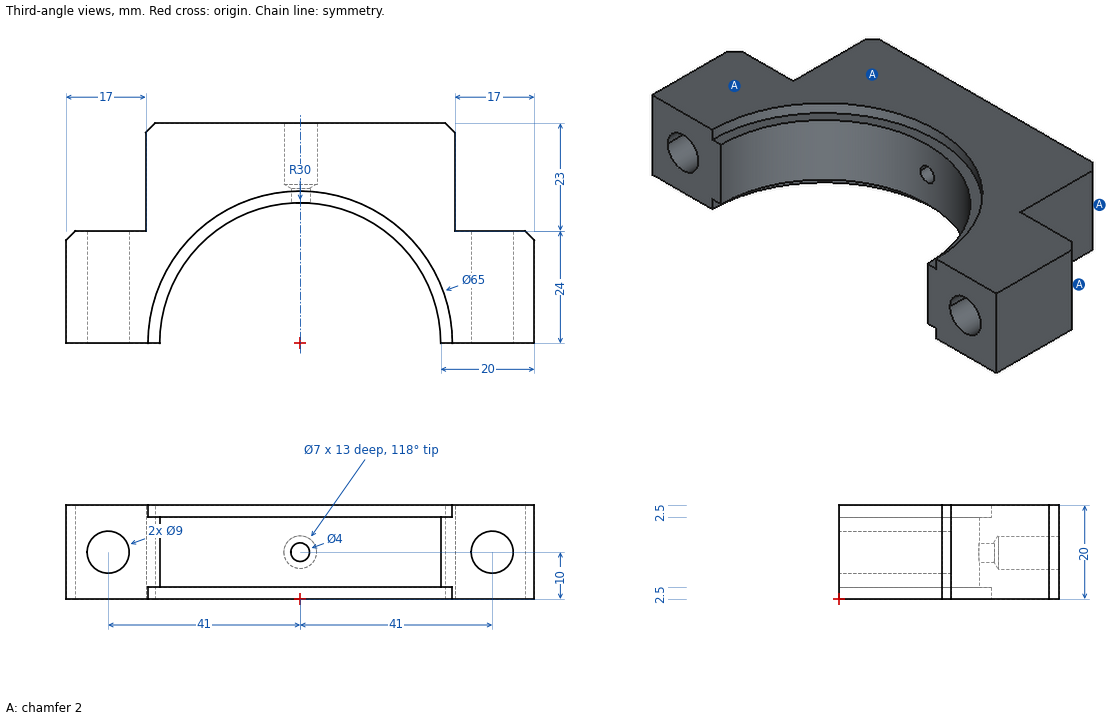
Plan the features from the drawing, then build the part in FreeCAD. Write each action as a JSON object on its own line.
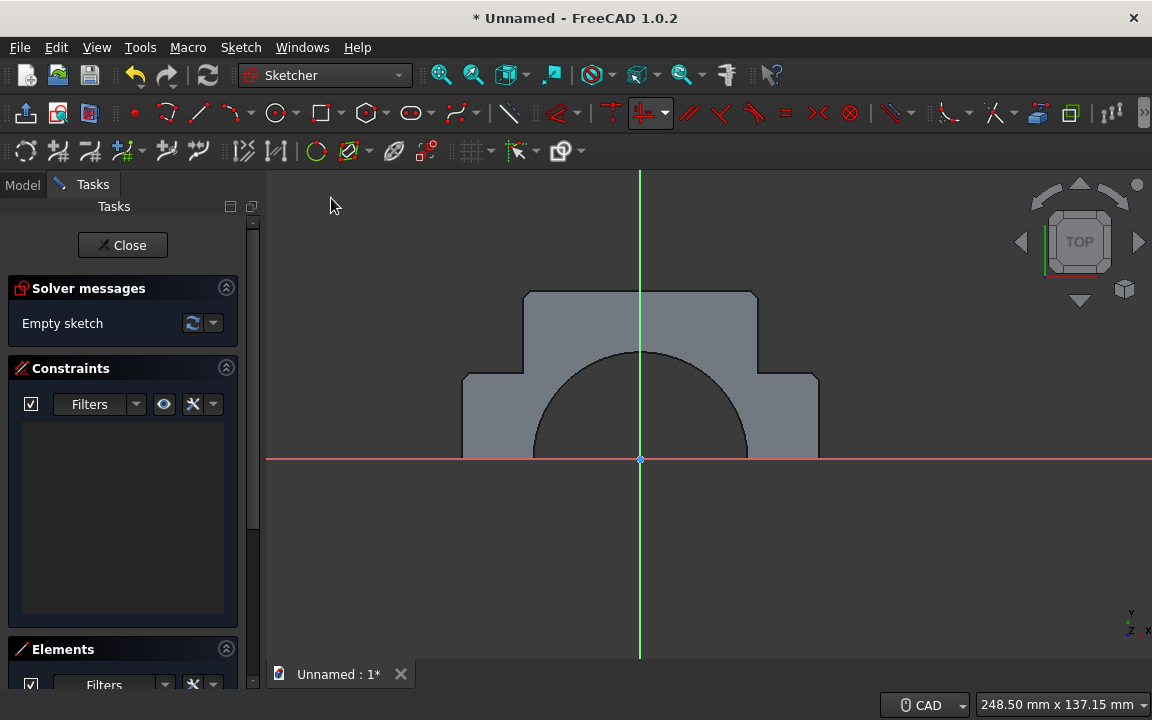
{"action": "left_click", "coordinate": [276, 114]}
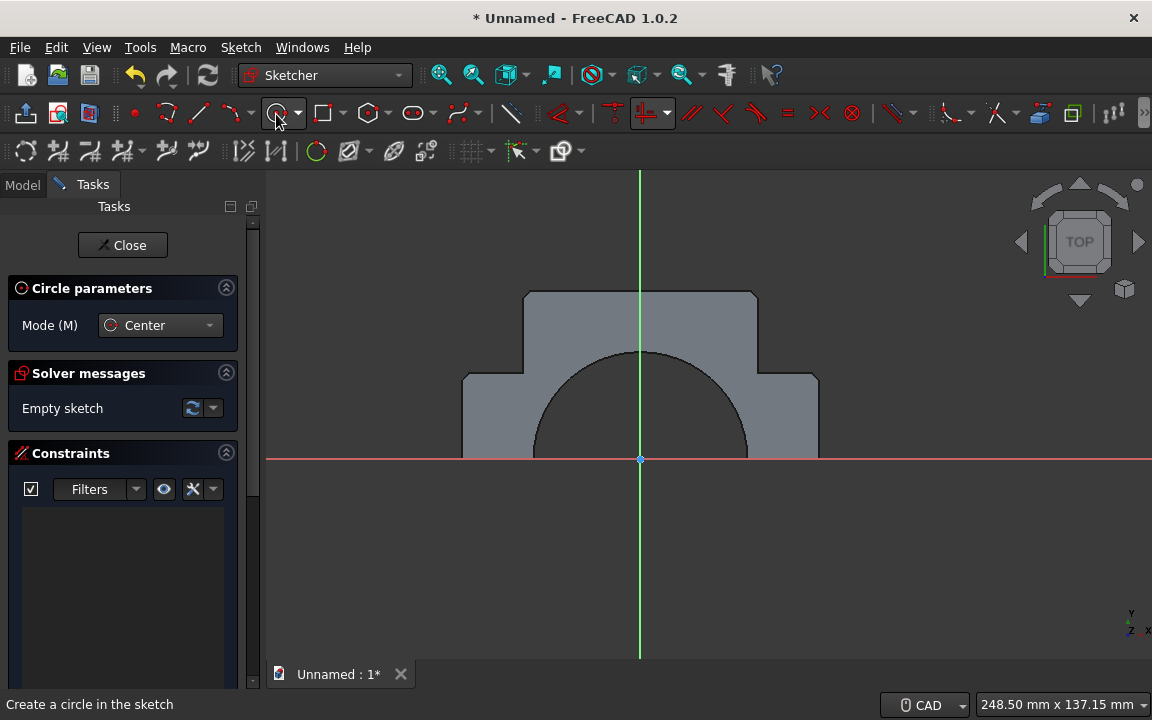
{"action": "left_click", "coordinate": [640, 459]}
{"action": "mouse_move", "coordinate": [722, 377]}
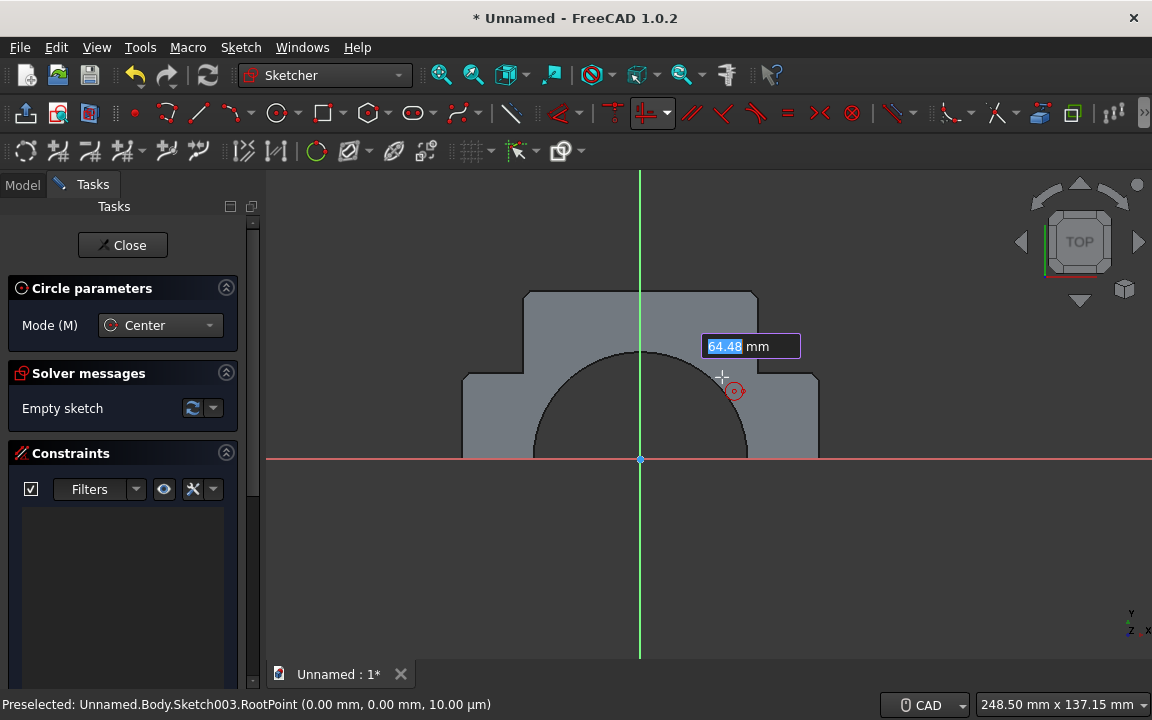
{"action": "type", "text": "65"}
{"action": "key", "text": "Return"}
{"action": "key", "text": "Escape"}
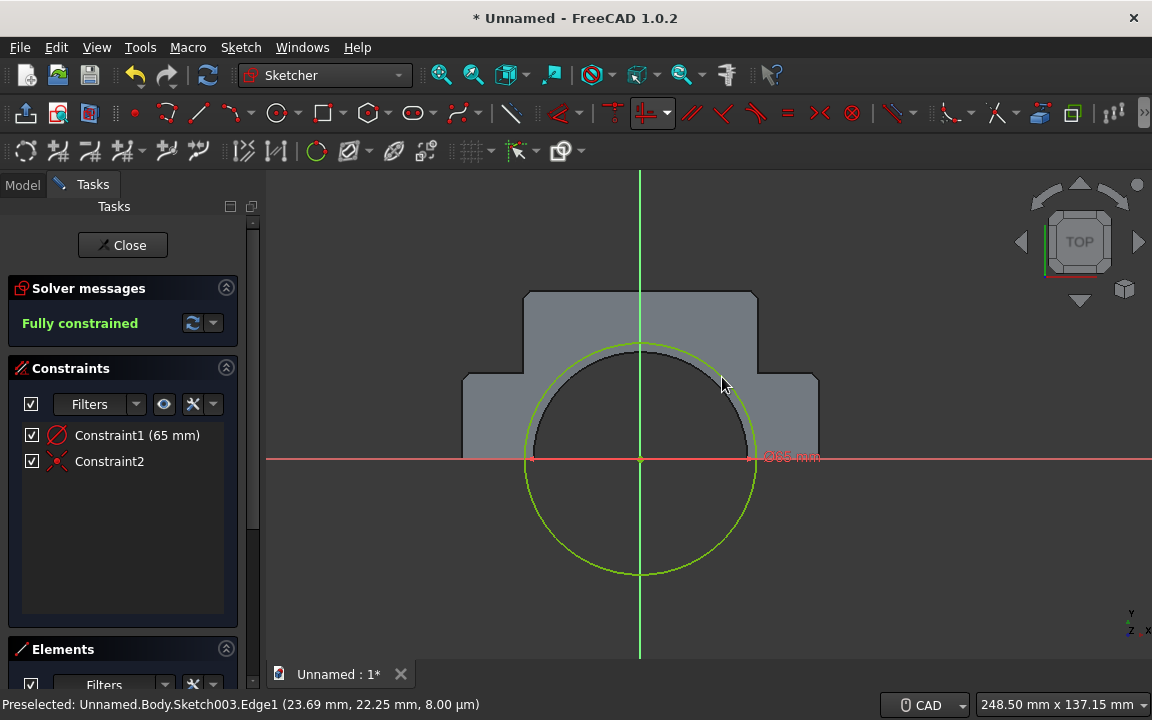
{"action": "left_click", "coordinate": [123, 245]}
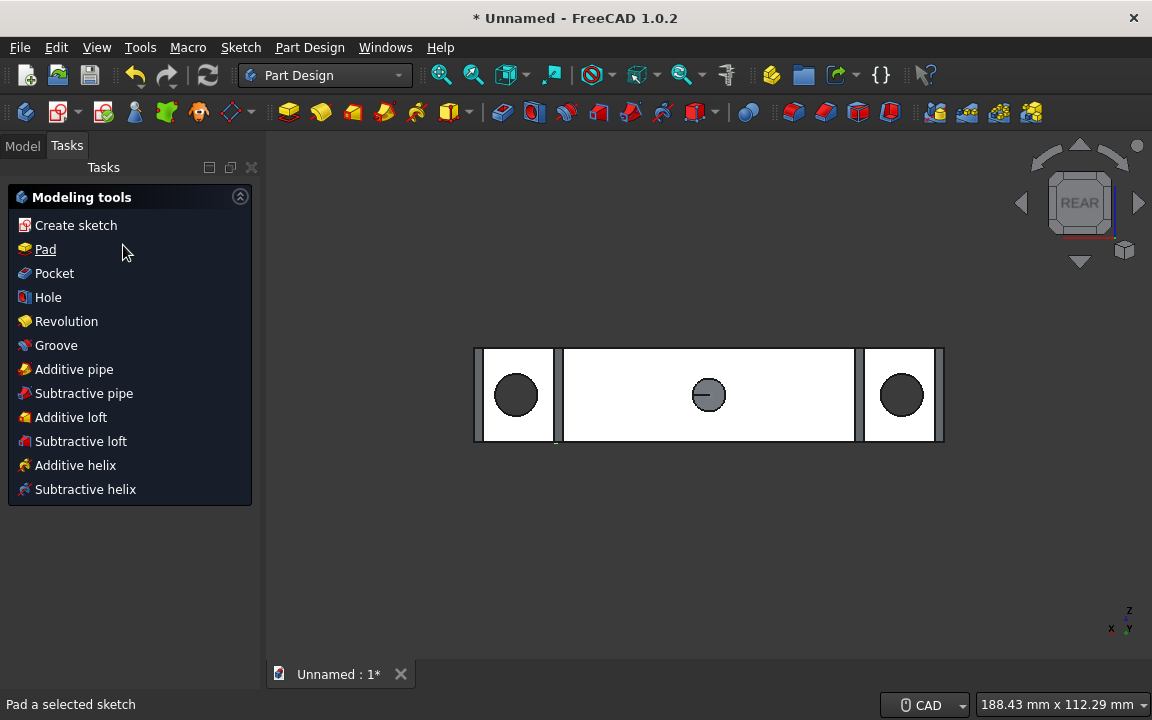
{"action": "left_click", "coordinate": [504, 112]}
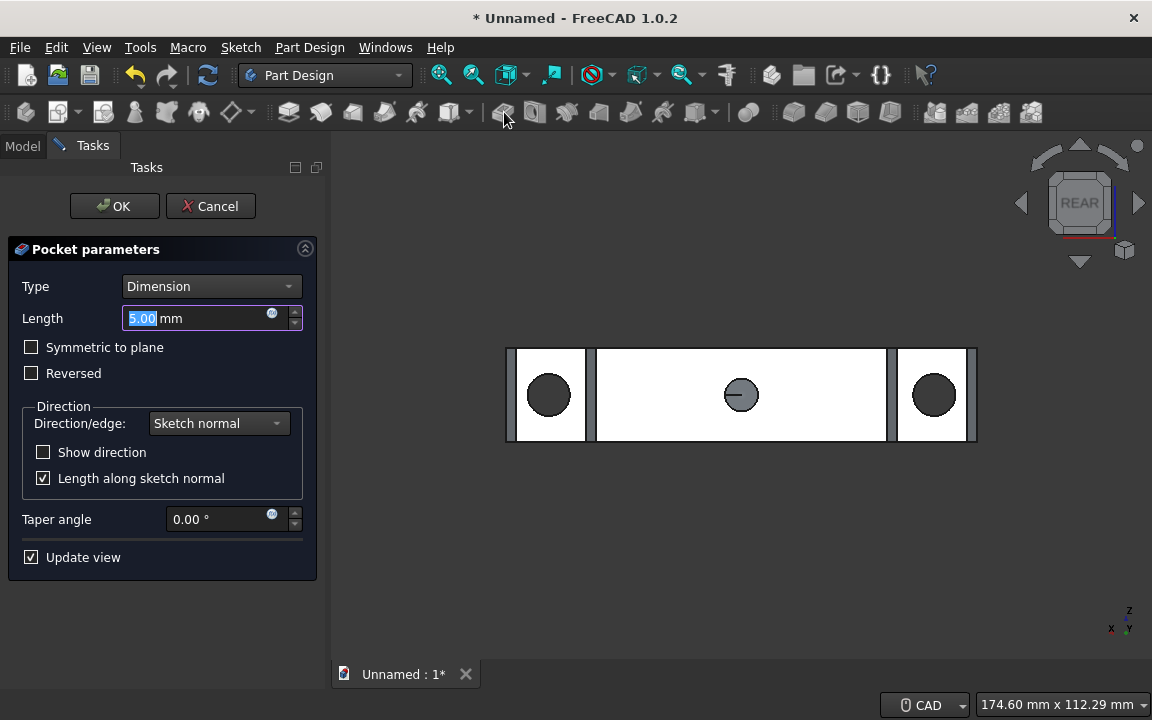
{"action": "type", "text": "2.5"}
{"action": "key", "text": "Tab"}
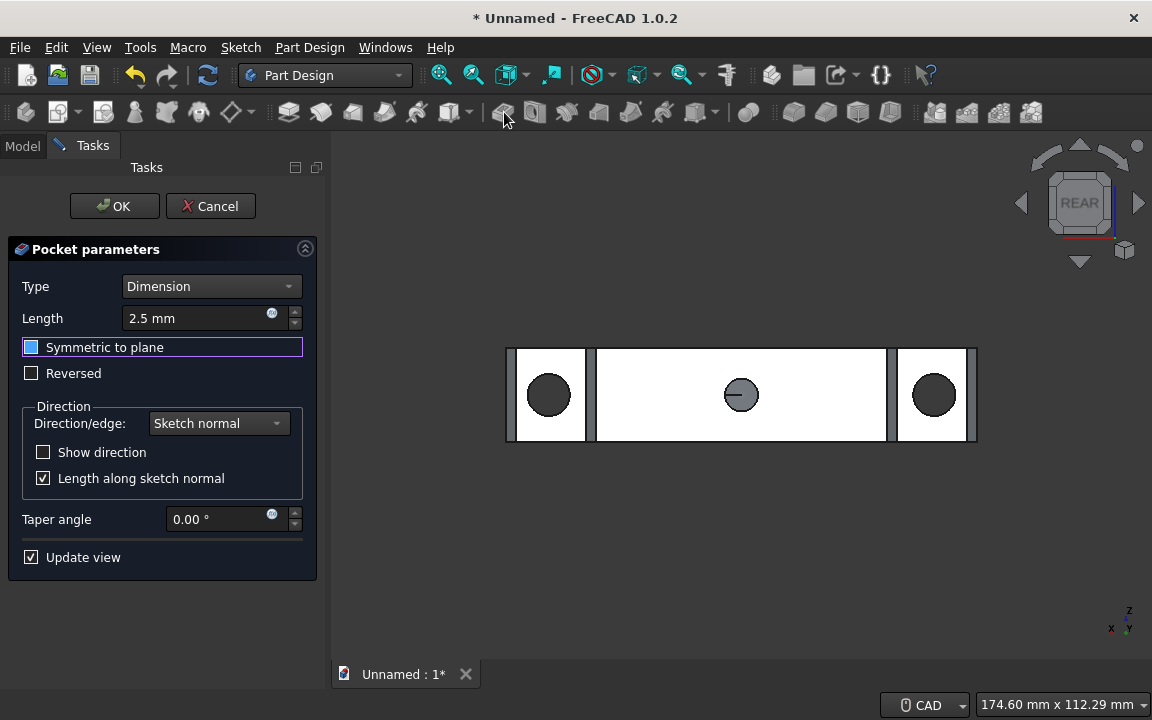
{"action": "left_click", "coordinate": [30, 373]}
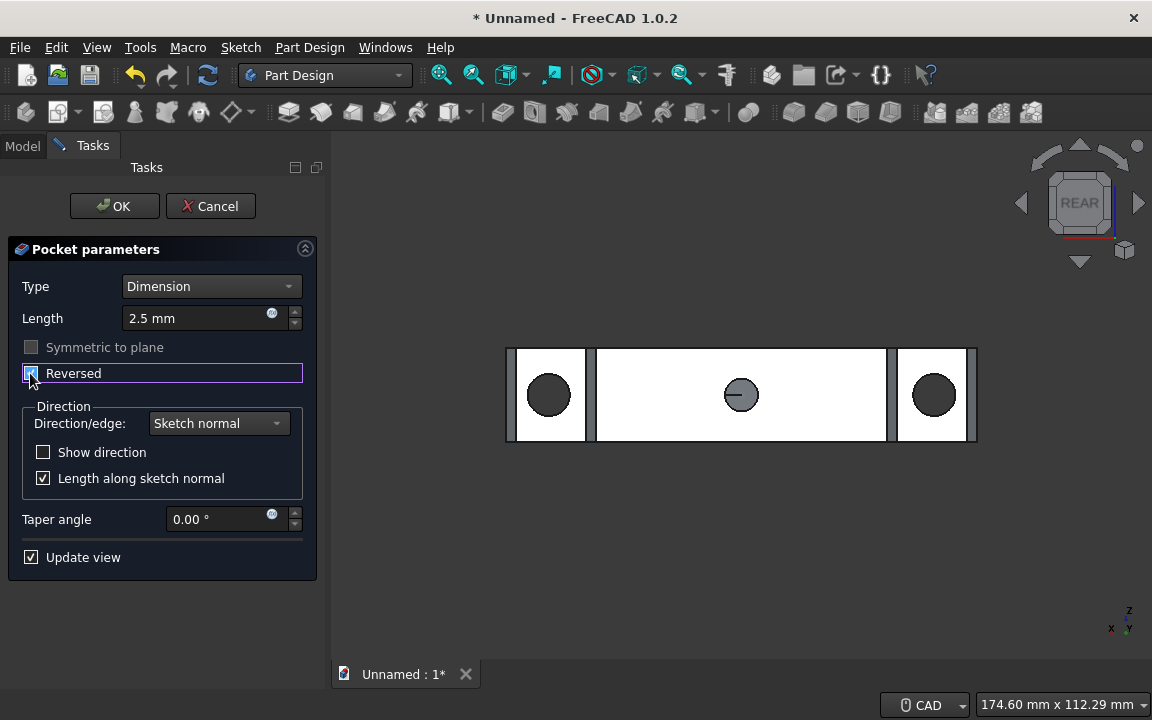
{"action": "left_click", "coordinate": [115, 206]}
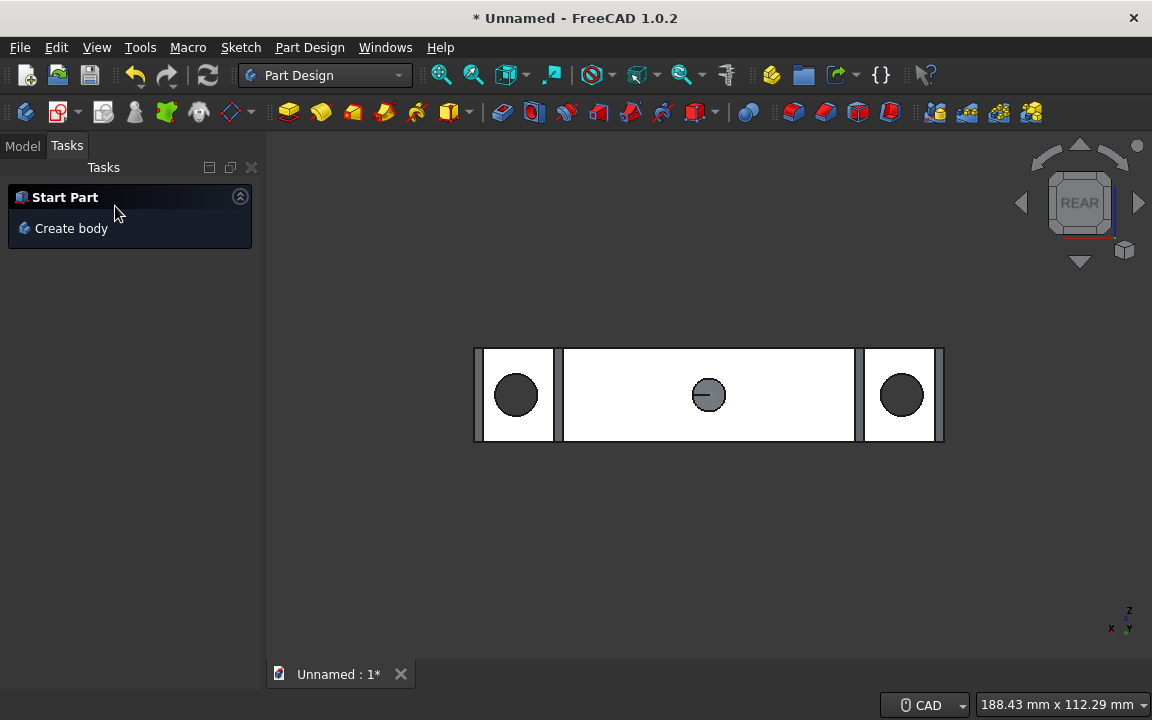
{"action": "left_click", "coordinate": [23, 145]}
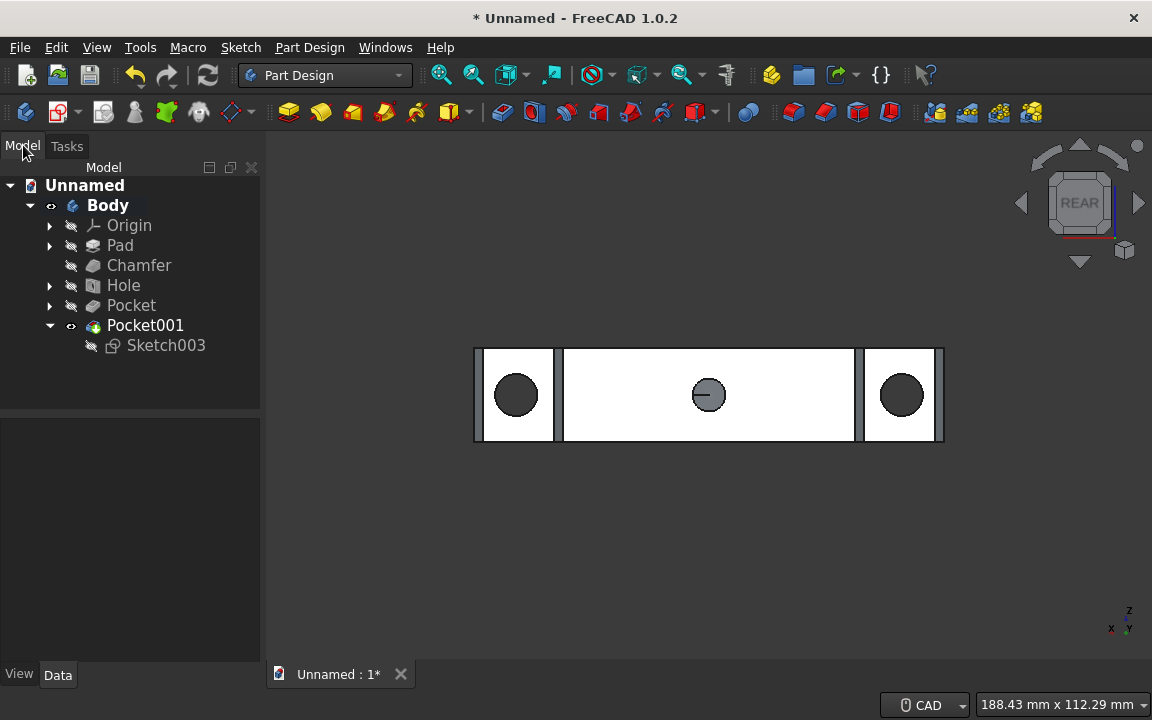
{"action": "left_click", "coordinate": [50, 226]}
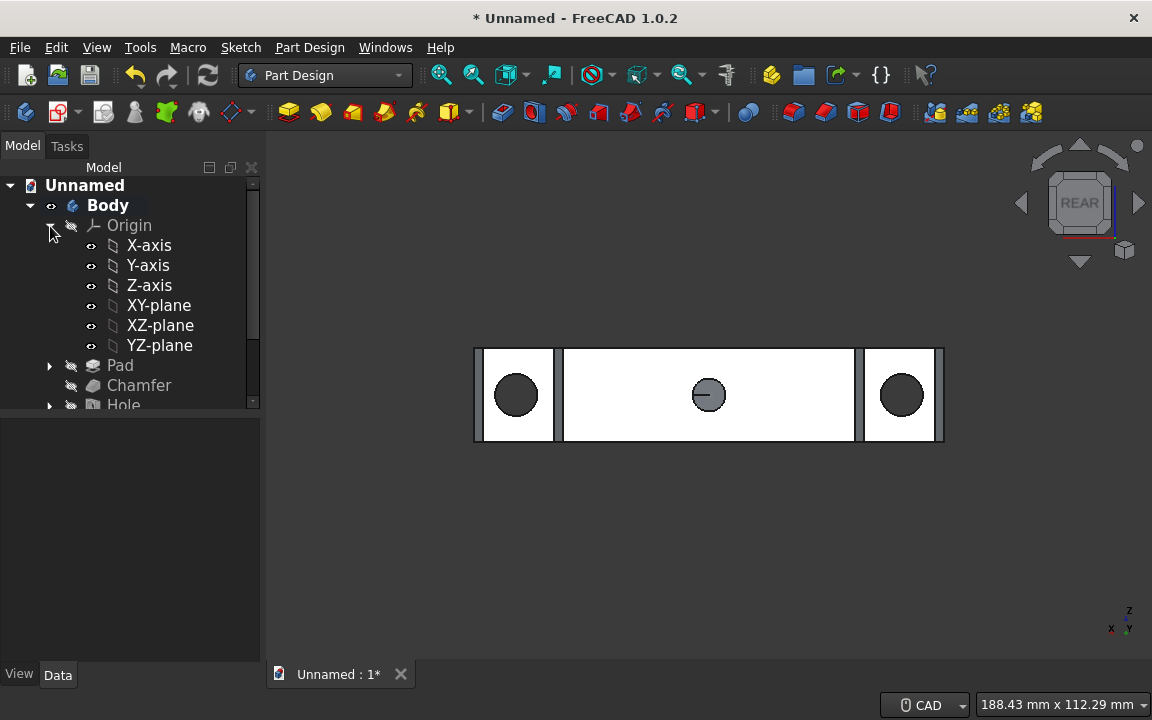
{"action": "left_click", "coordinate": [136, 306]}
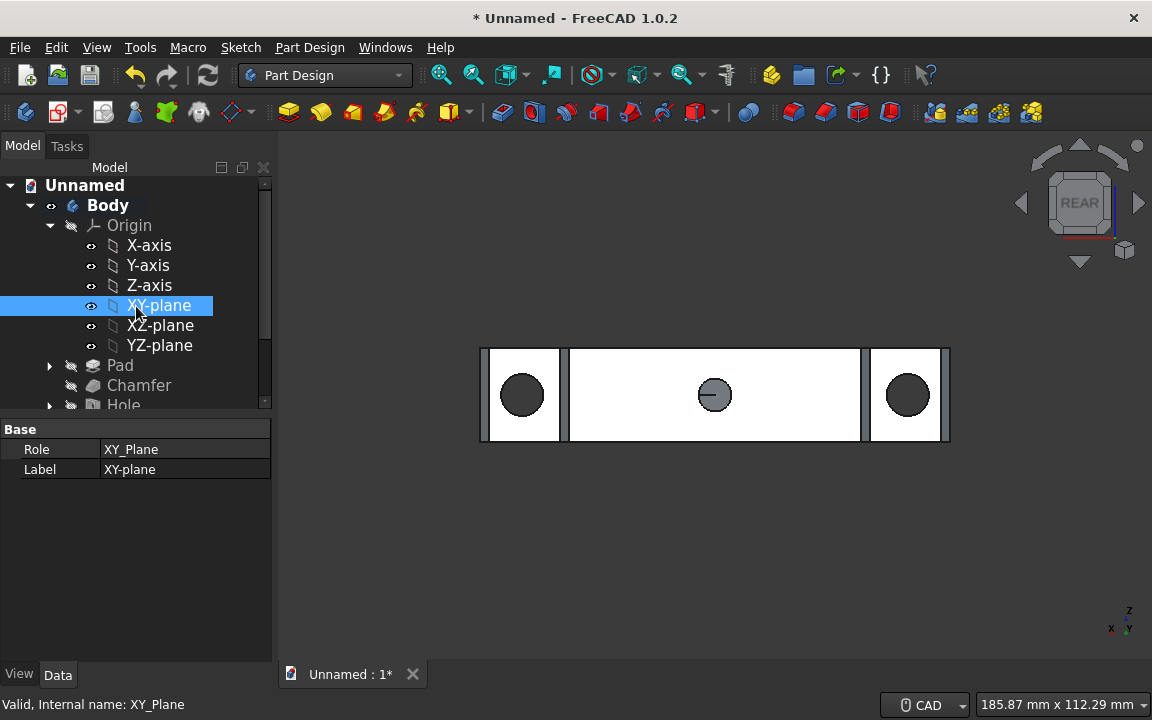
{"action": "left_click", "coordinate": [232, 112]}